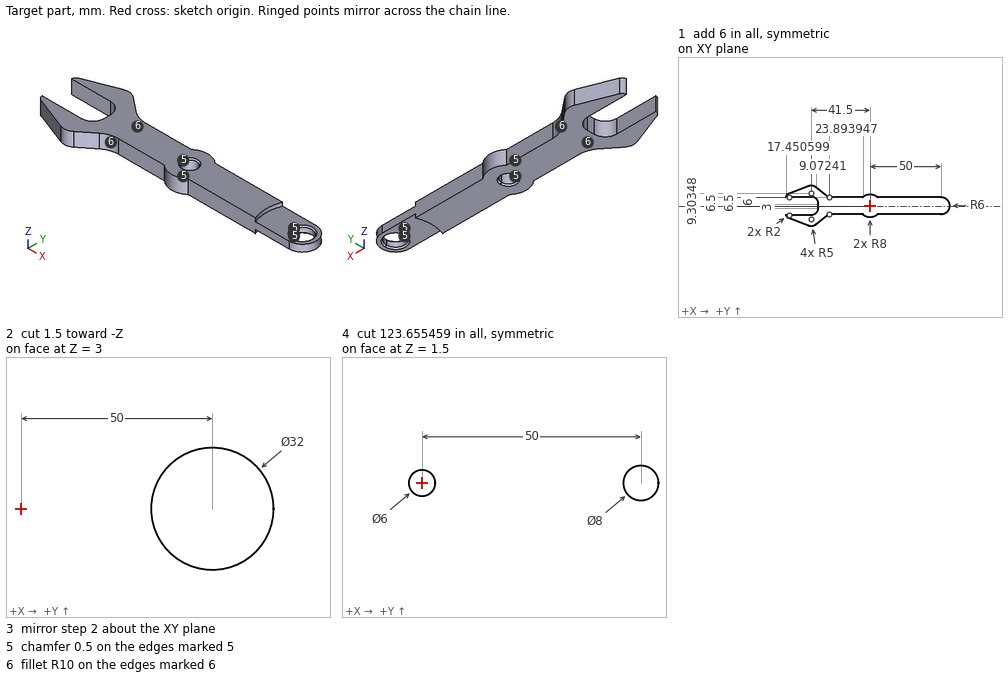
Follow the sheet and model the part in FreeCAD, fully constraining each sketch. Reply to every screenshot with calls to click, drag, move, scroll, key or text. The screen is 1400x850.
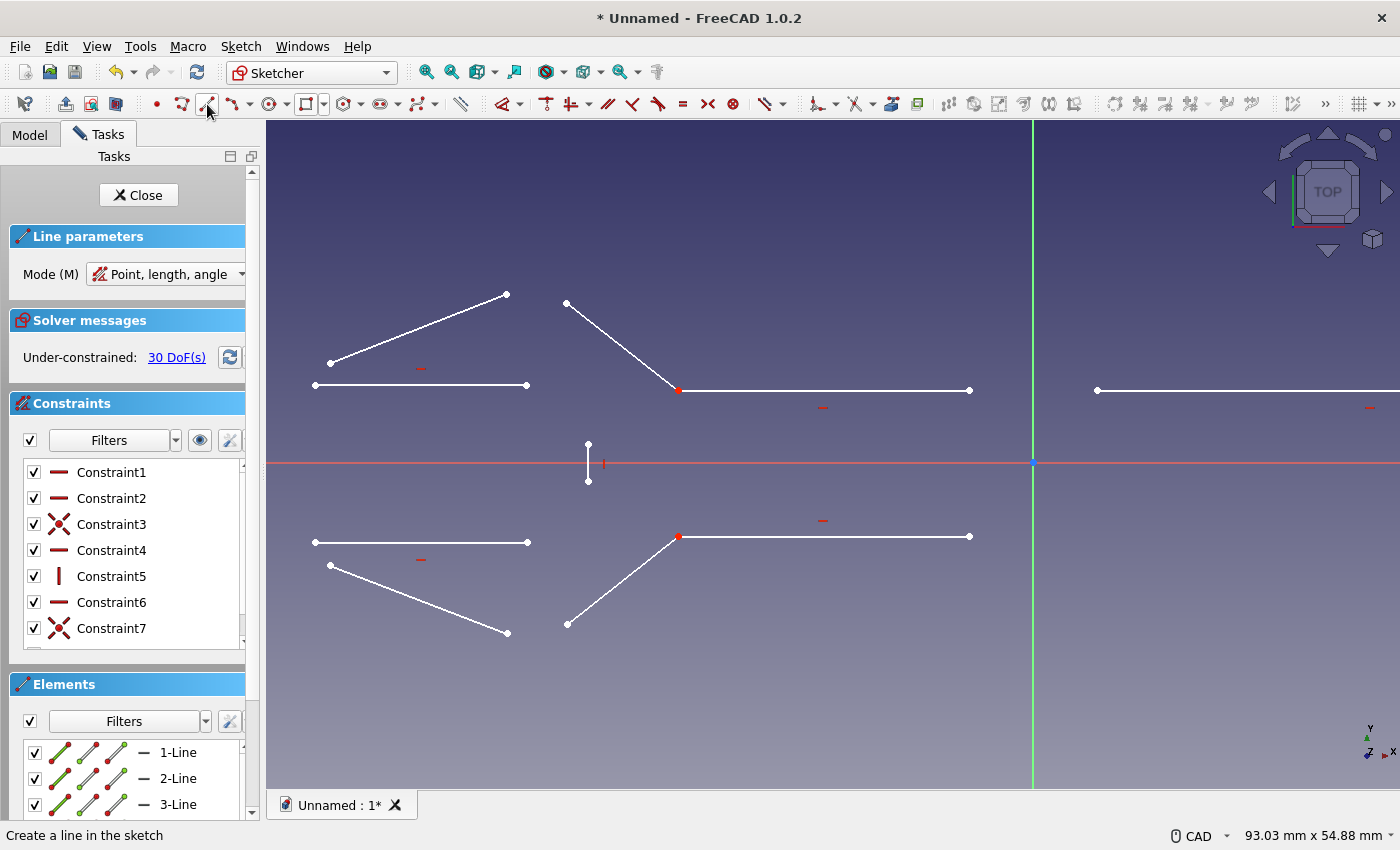
click(1098, 536)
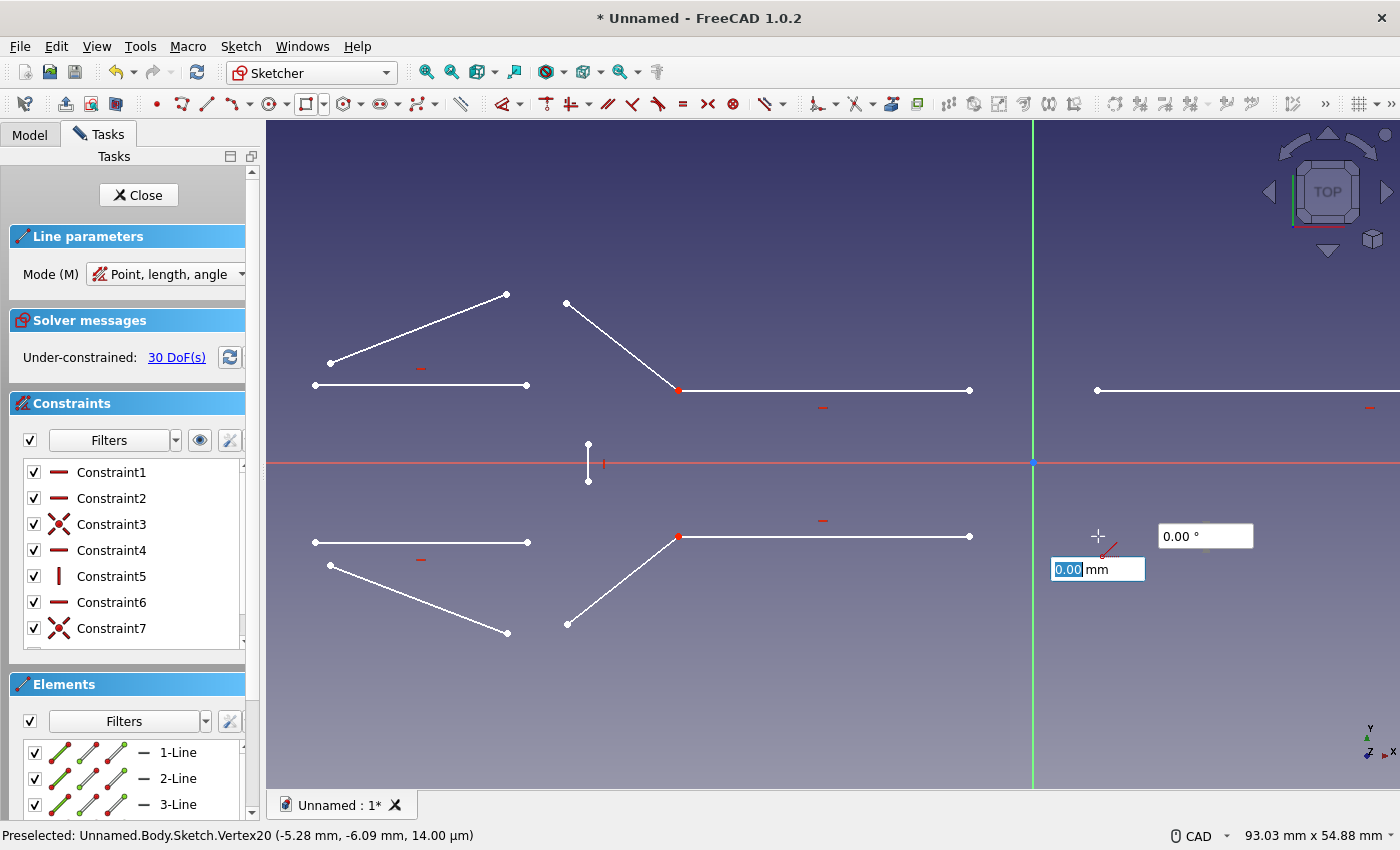
scroll(560, 448, down, 4)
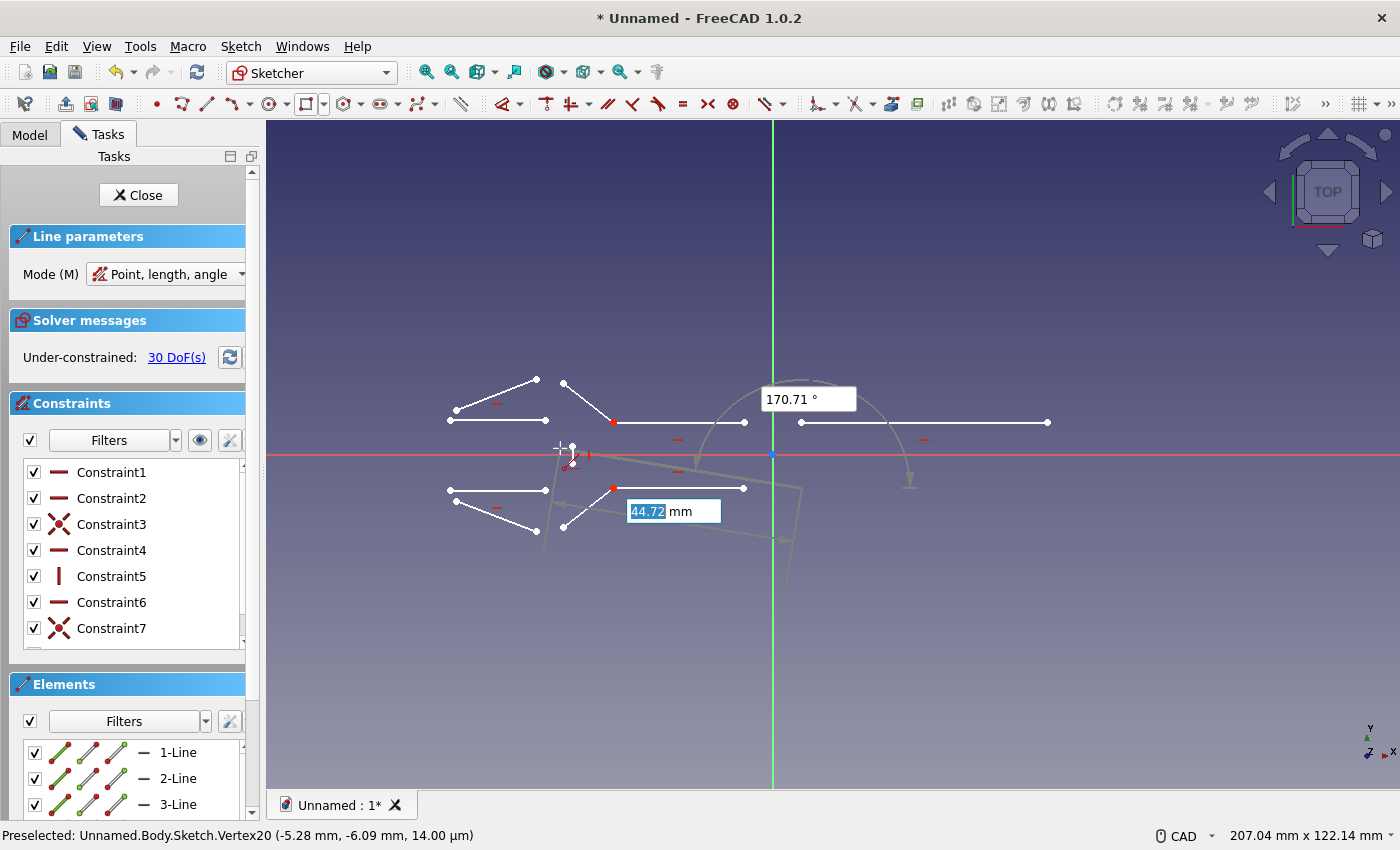
click(1047, 488)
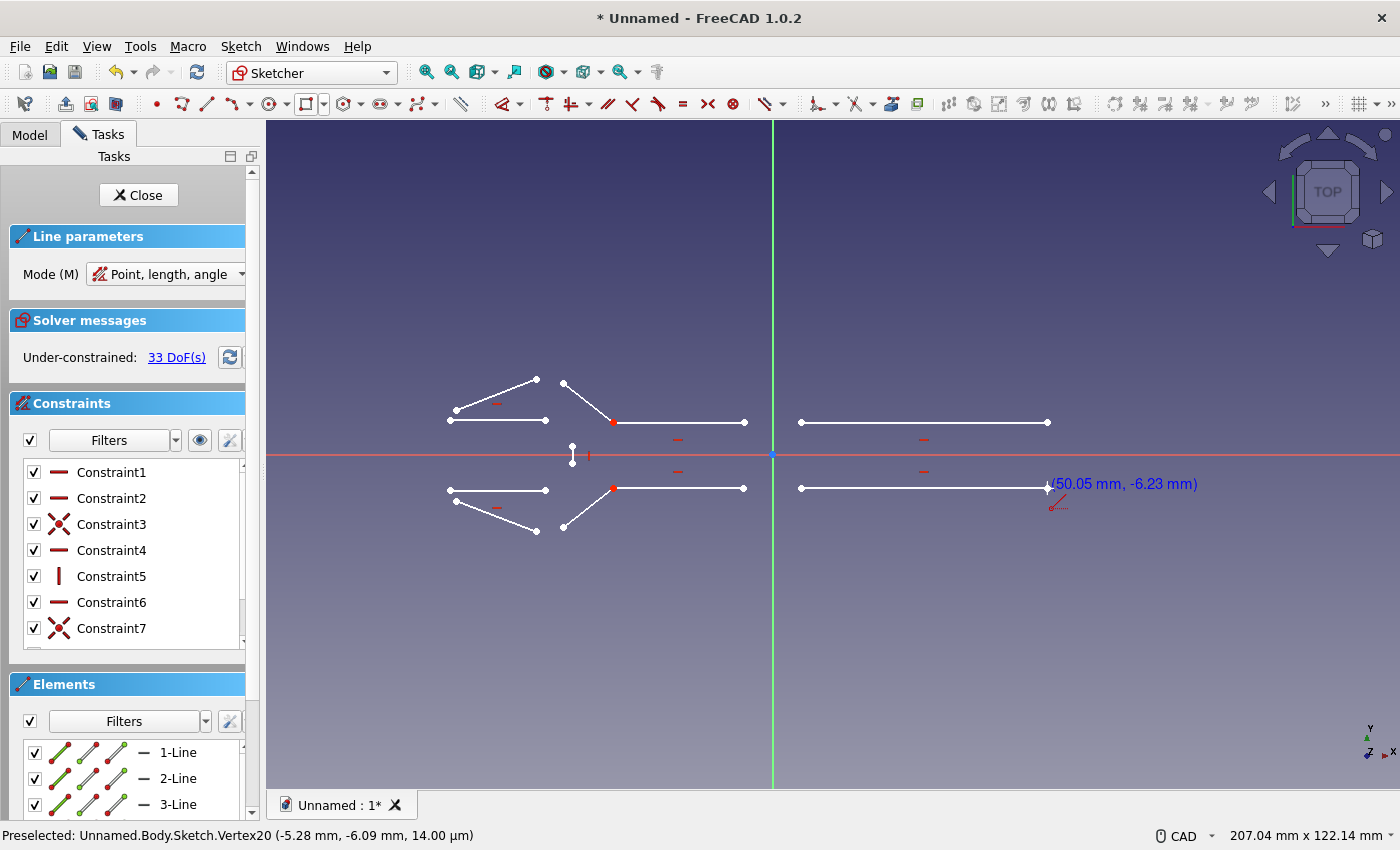
click(232, 104)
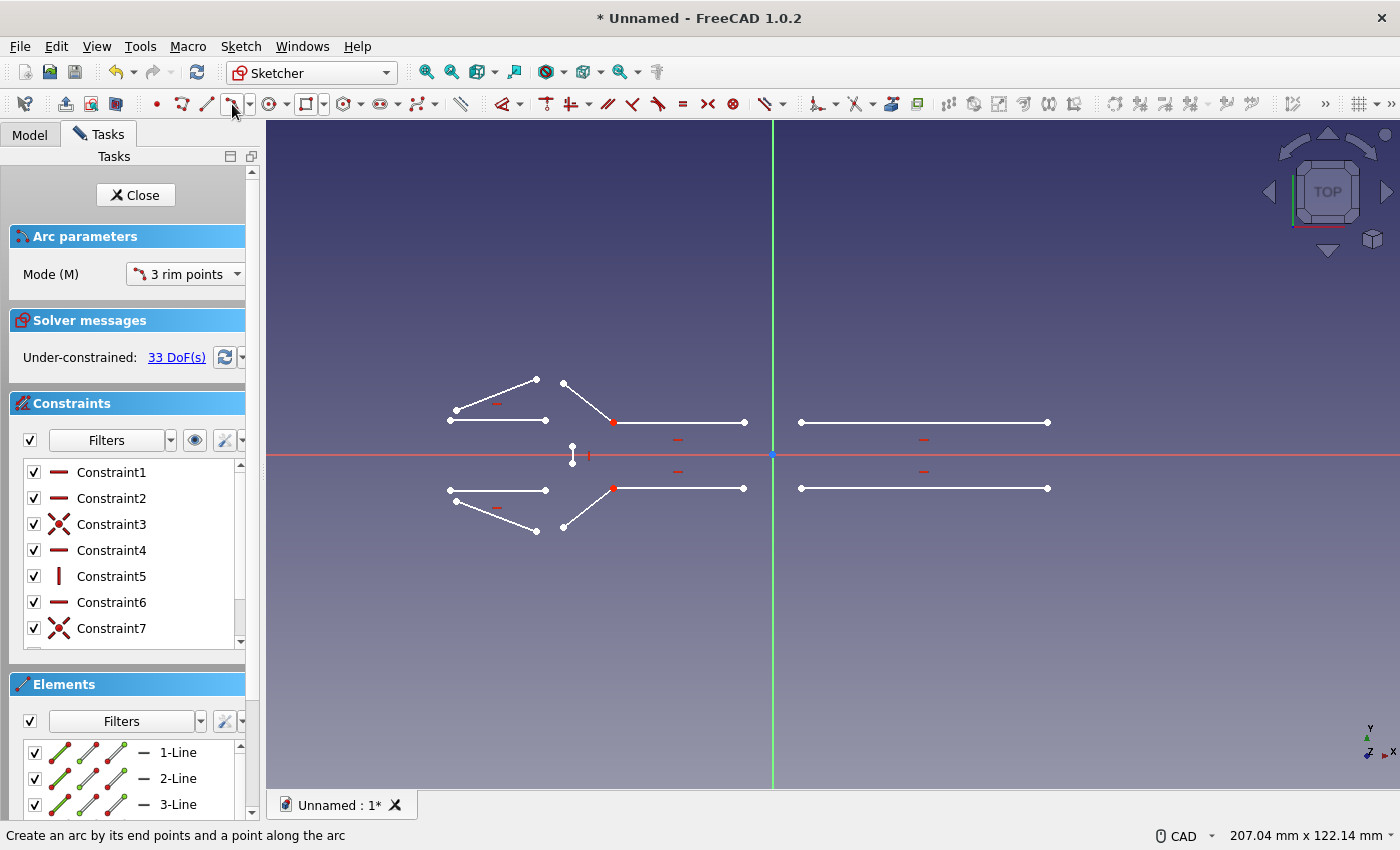
click(801, 423)
click(744, 423)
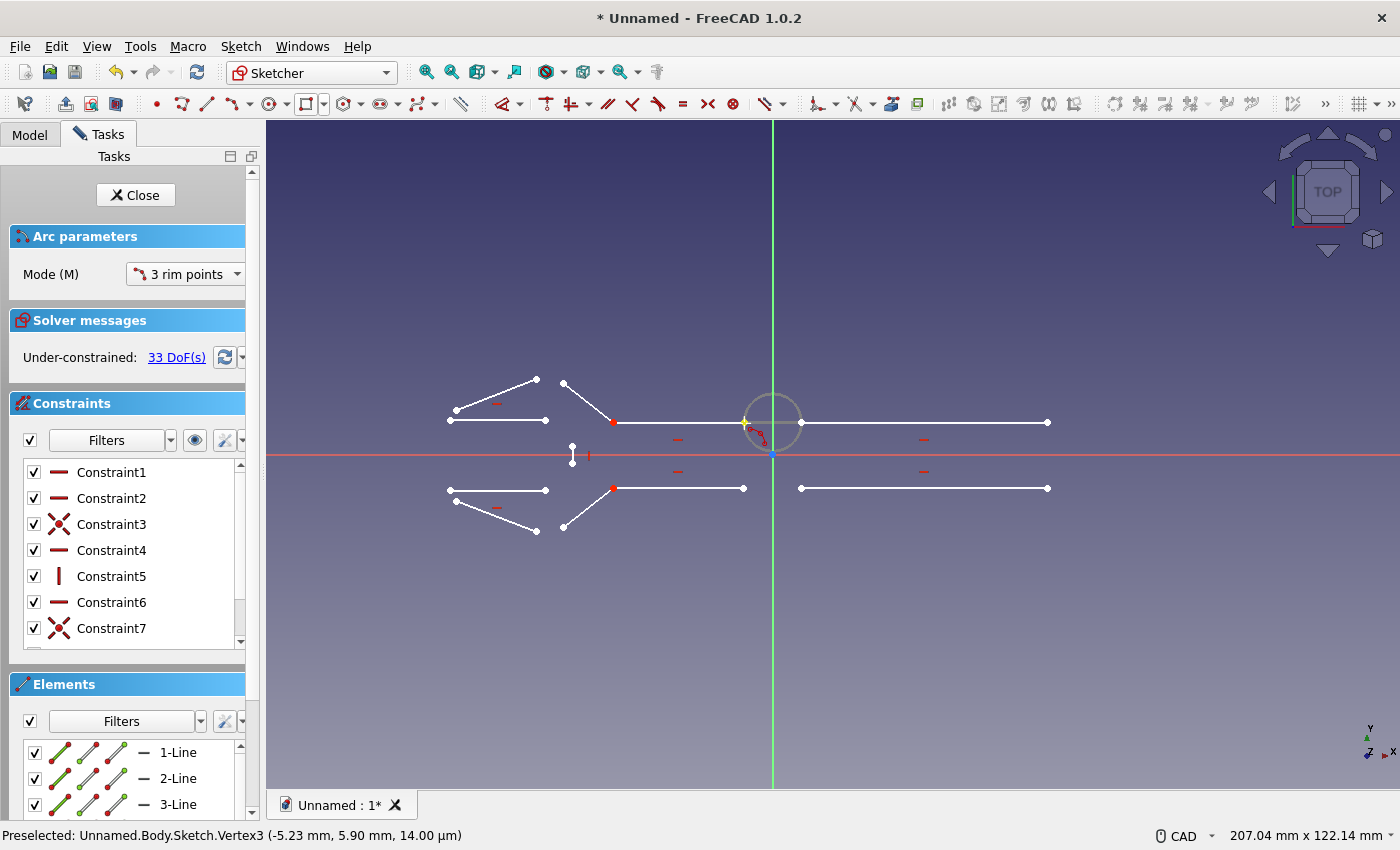
scroll(760, 413, up, 3)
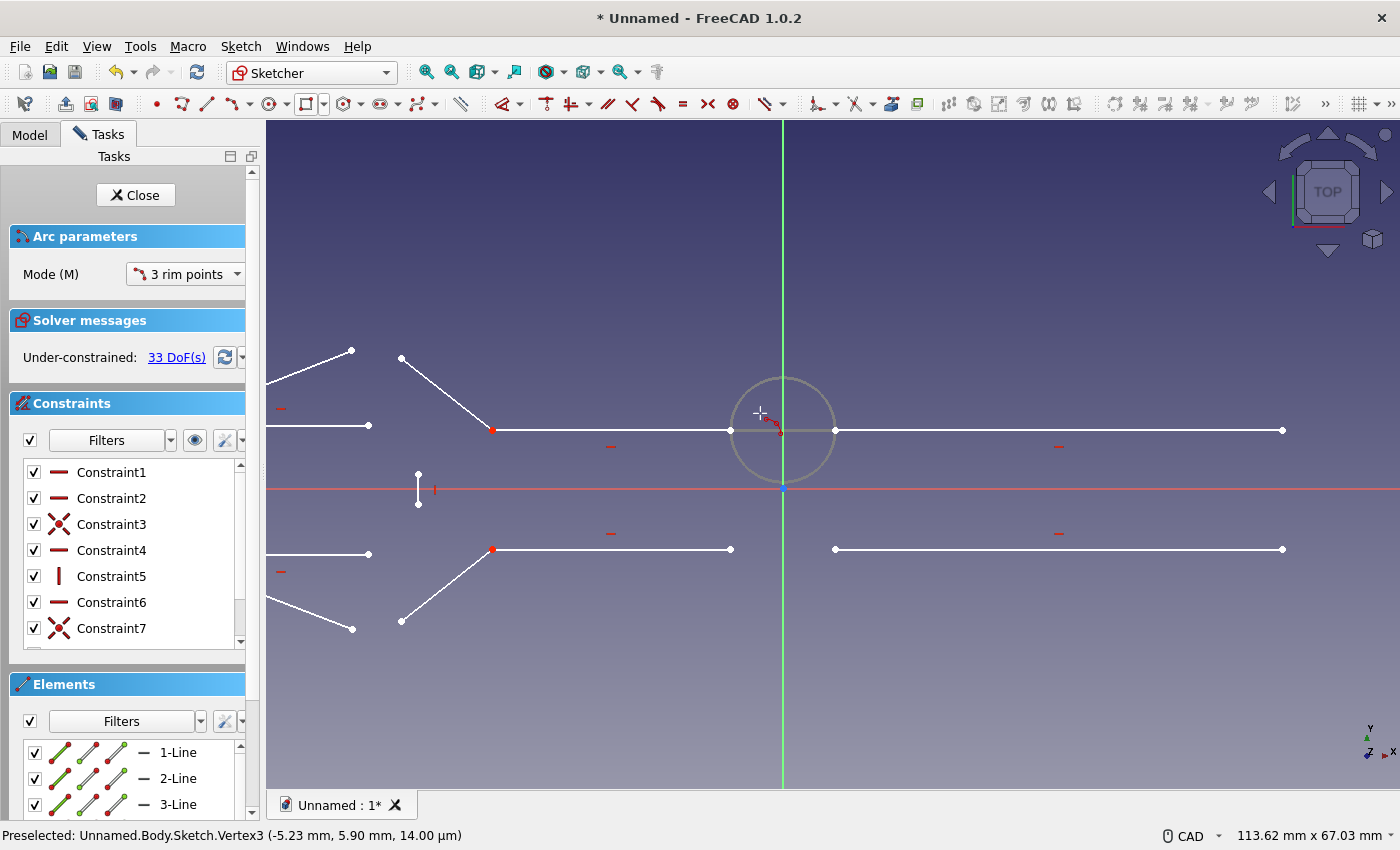
click(760, 412)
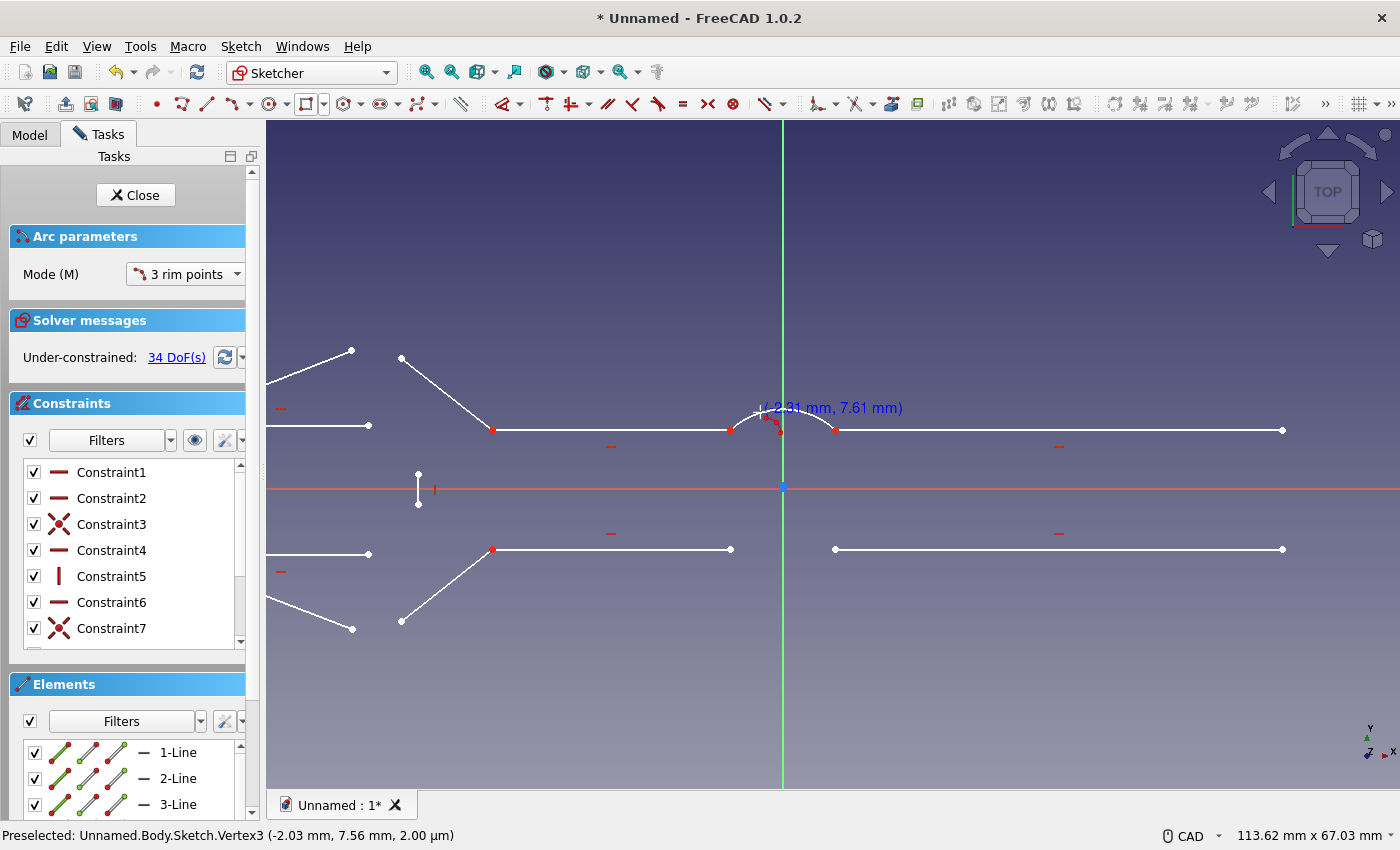
click(401, 358)
click(352, 351)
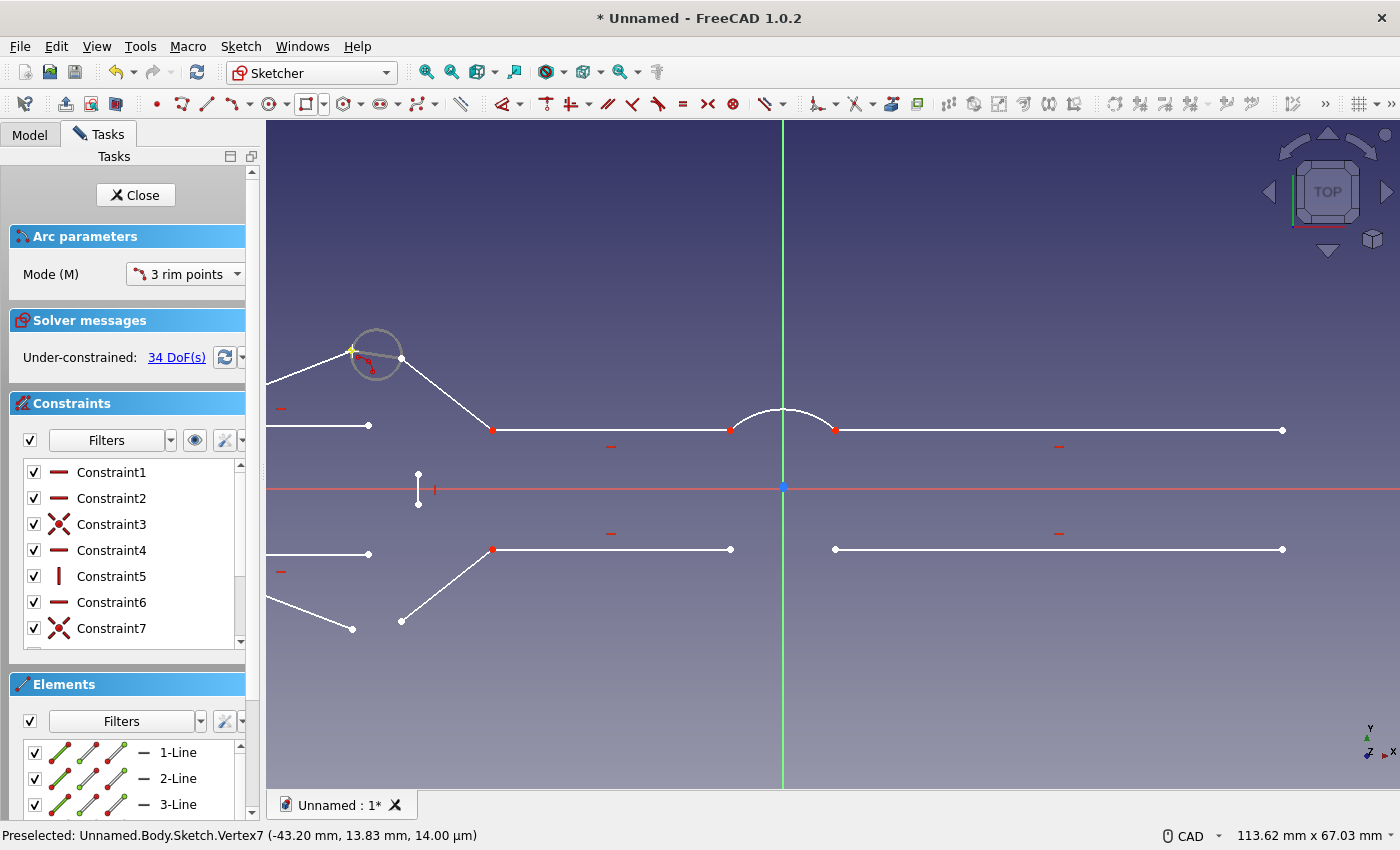
scroll(378, 347, up, 5)